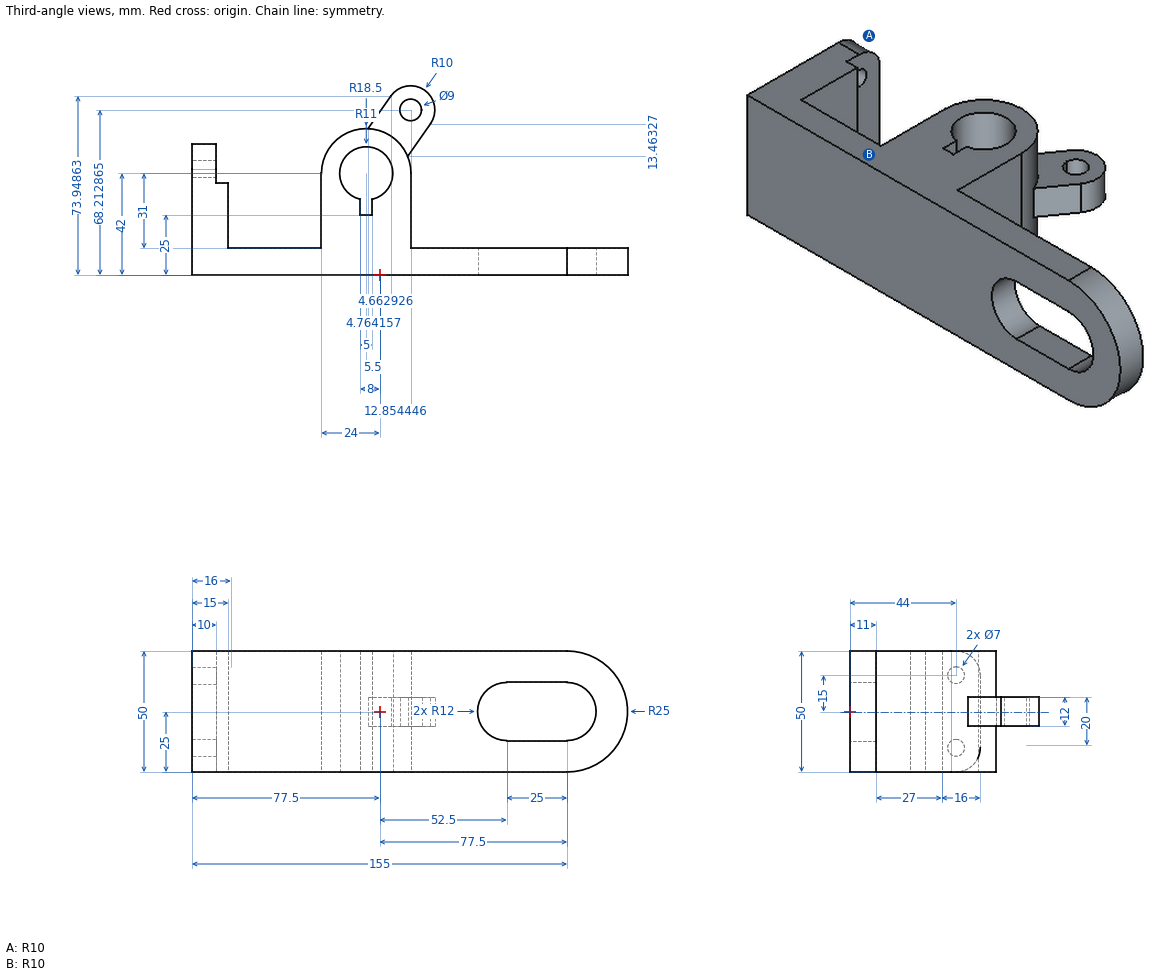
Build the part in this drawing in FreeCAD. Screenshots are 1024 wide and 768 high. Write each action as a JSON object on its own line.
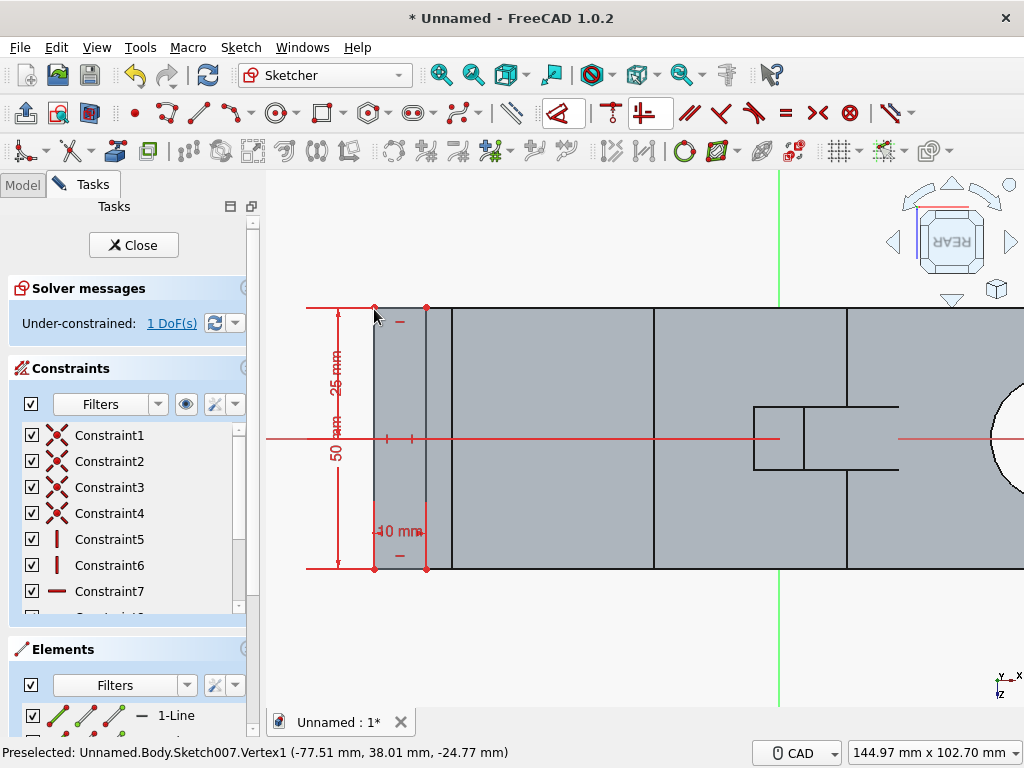
{"action": "left_click", "coordinate": [374, 308]}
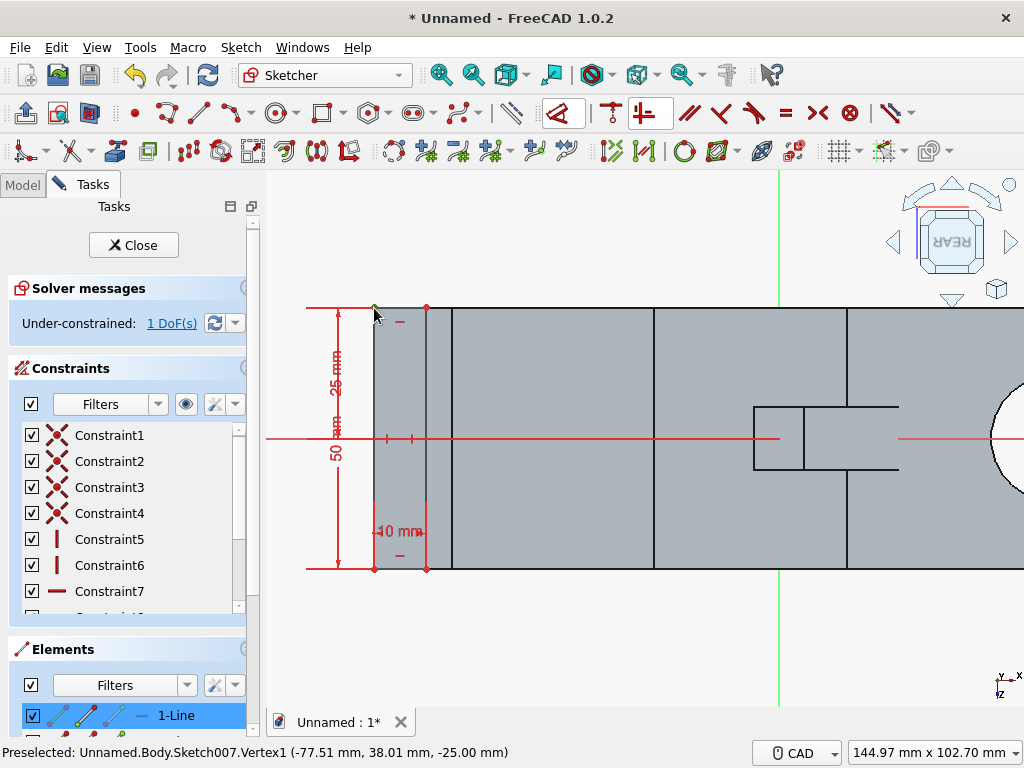
{"action": "key", "text": "l"}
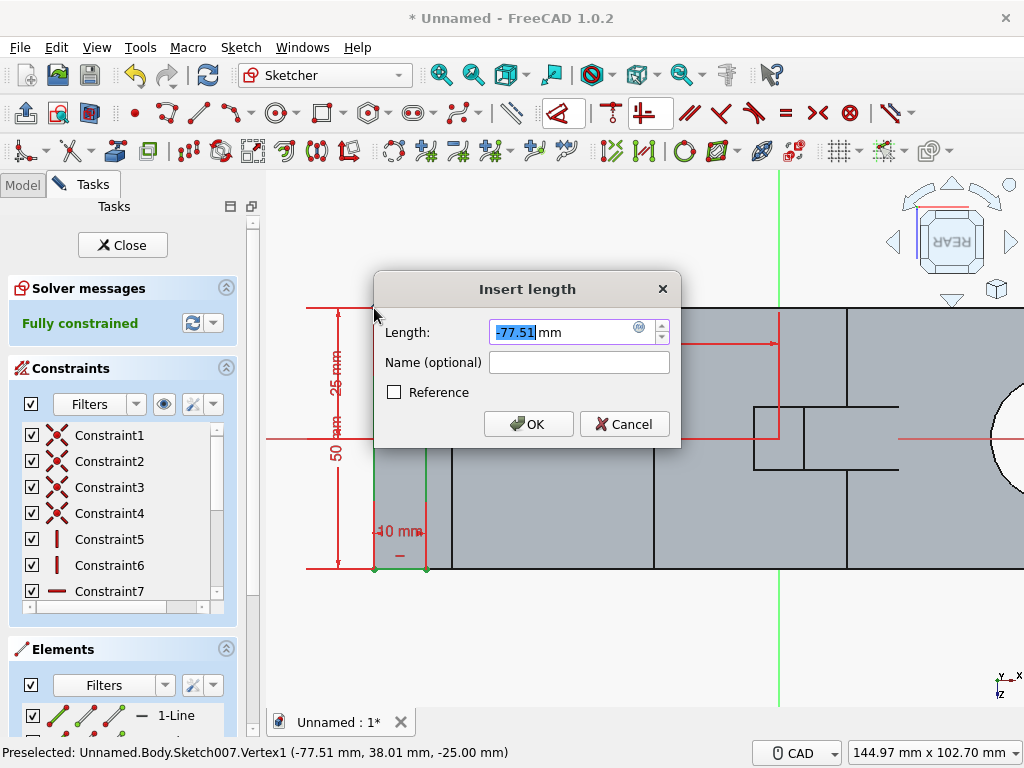
{"action": "type", "text": "-77.5"}
{"action": "key", "text": "Return"}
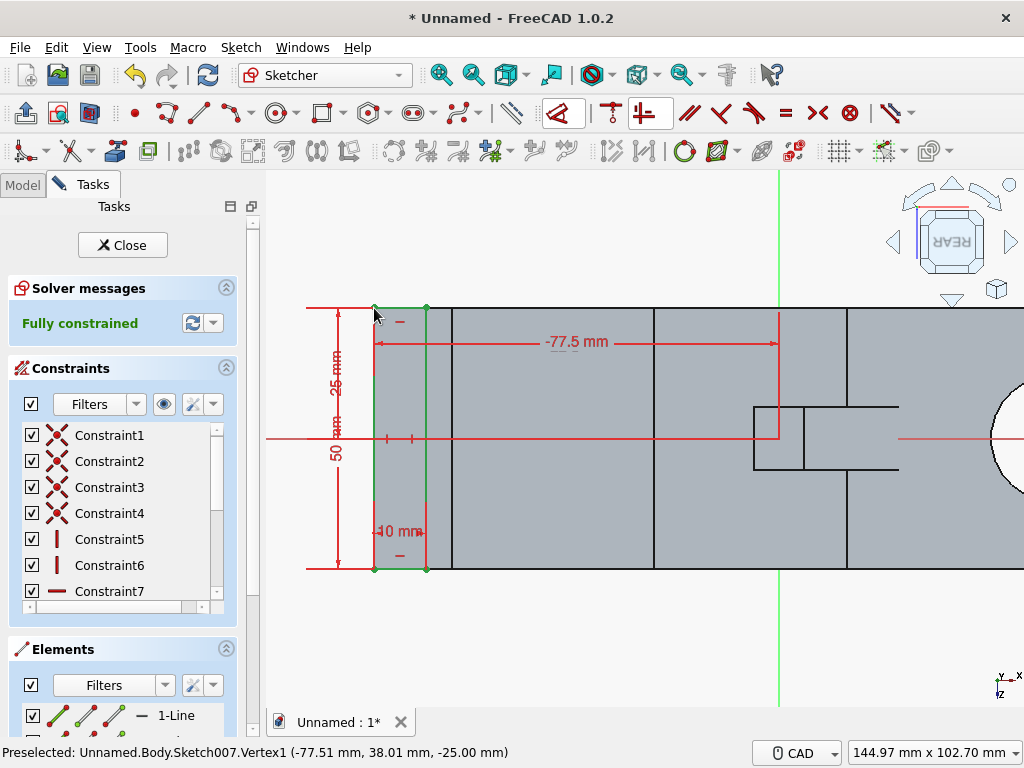
{"action": "left_click", "coordinate": [123, 245]}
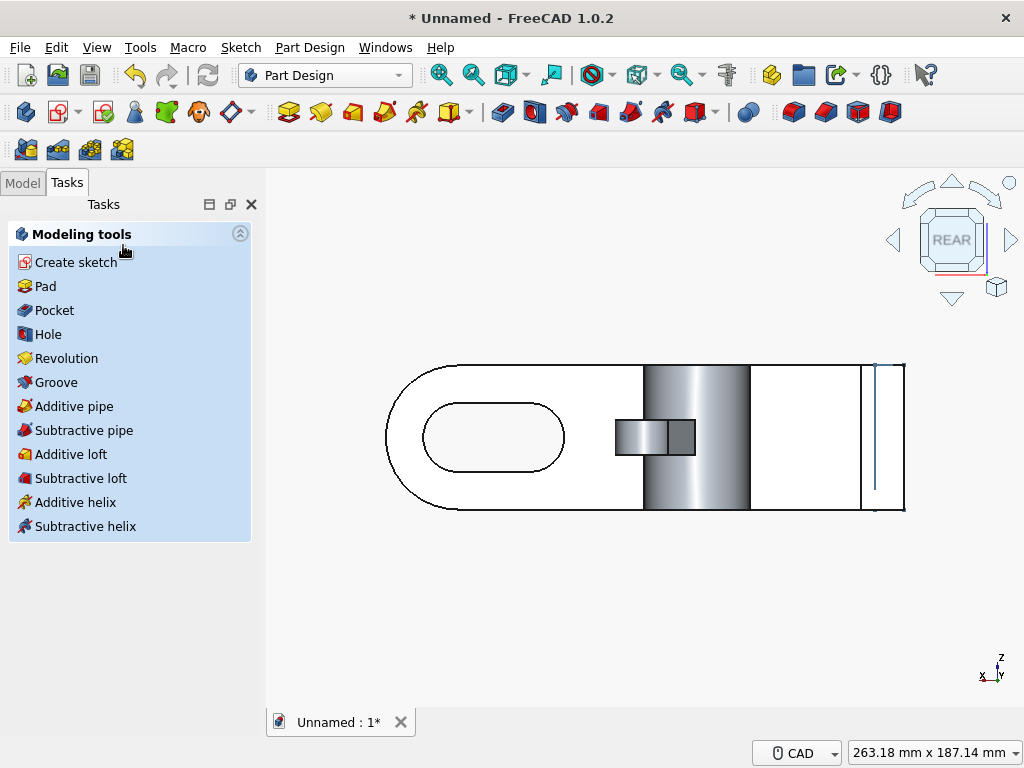
{"action": "left_click", "coordinate": [290, 112]}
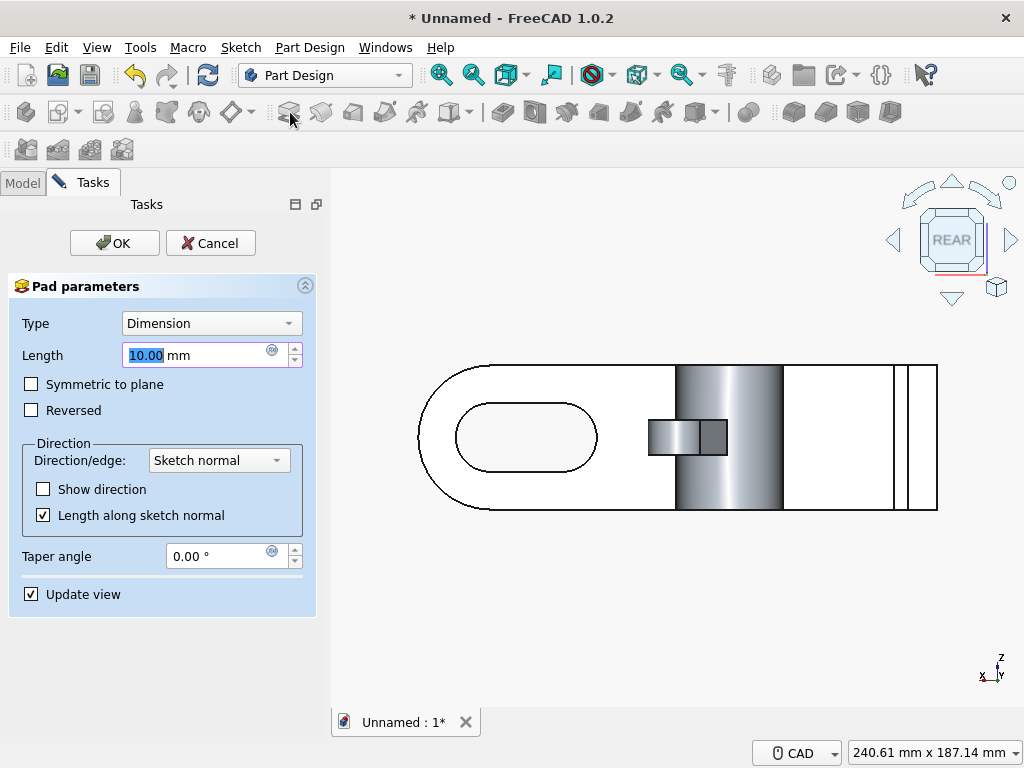
{"action": "type", "text": "16"}
{"action": "key", "text": "Tab"}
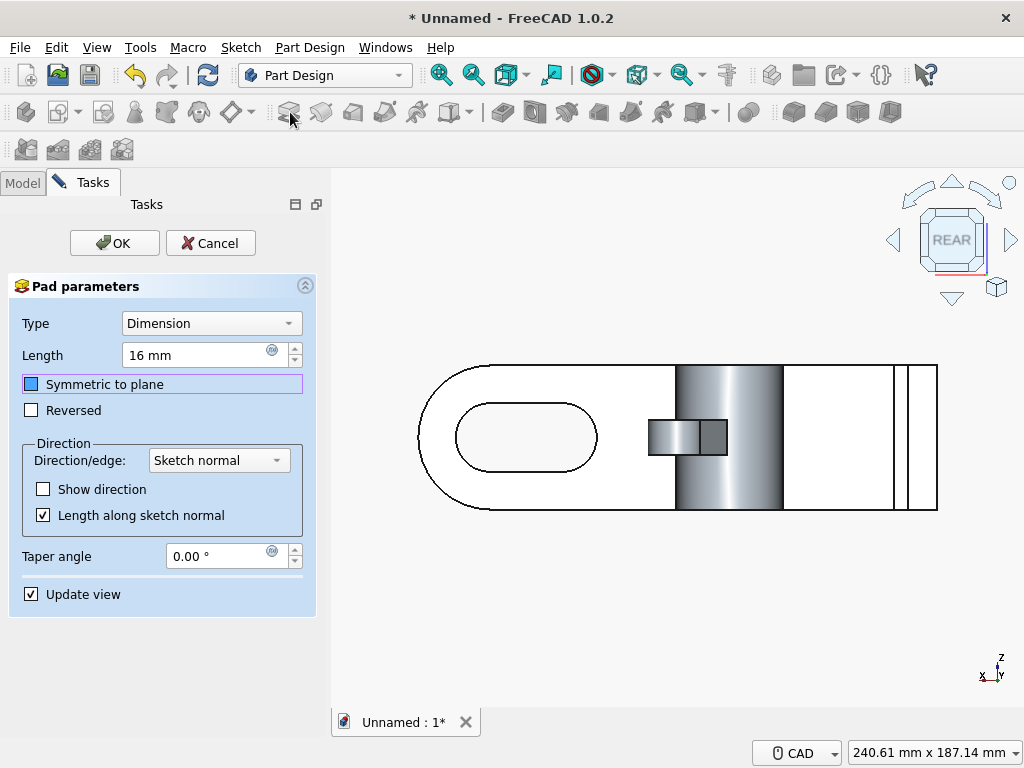
{"action": "left_click", "coordinate": [115, 243]}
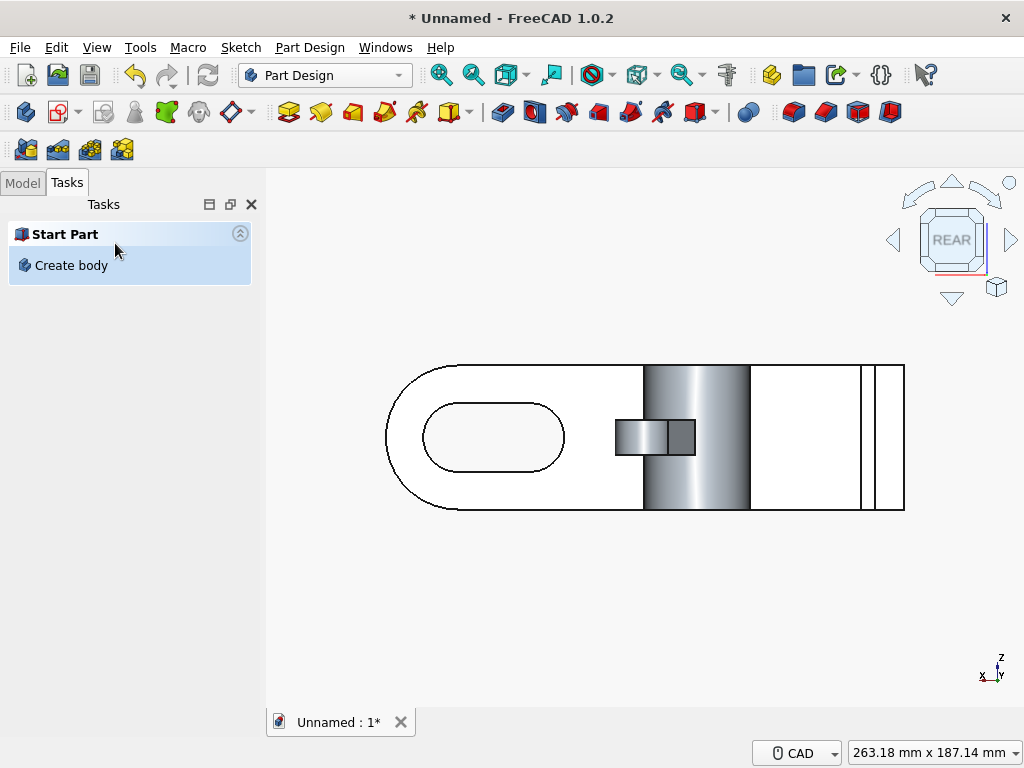
{"action": "key", "text": "0"}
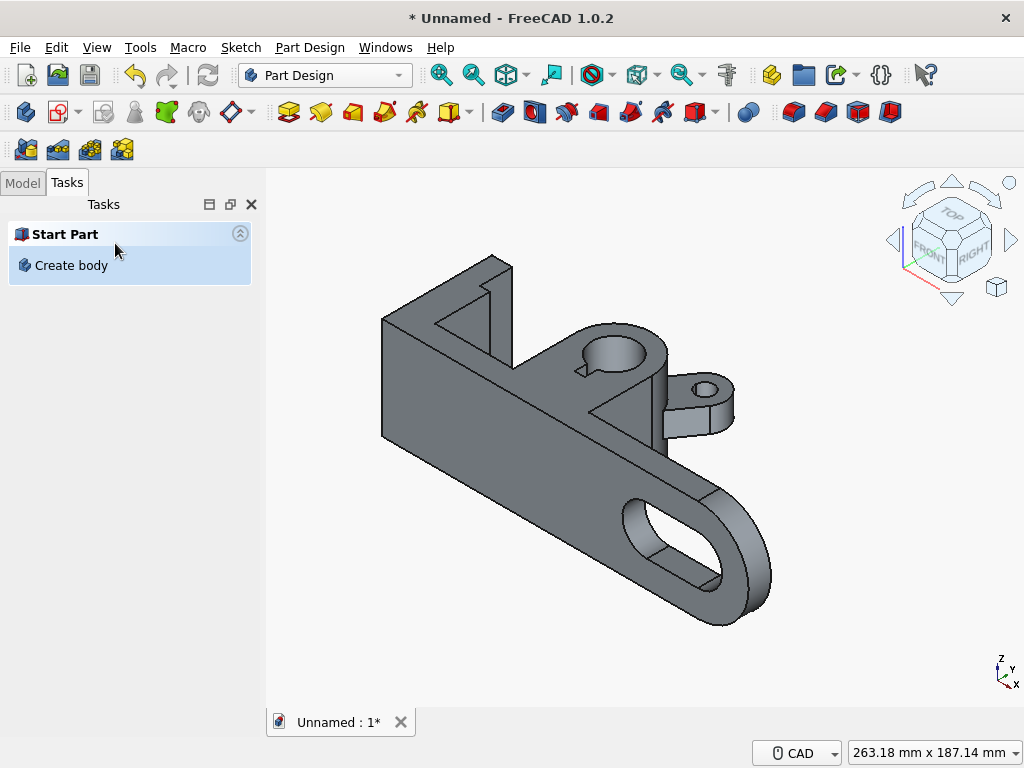
{"action": "key", "text": "2"}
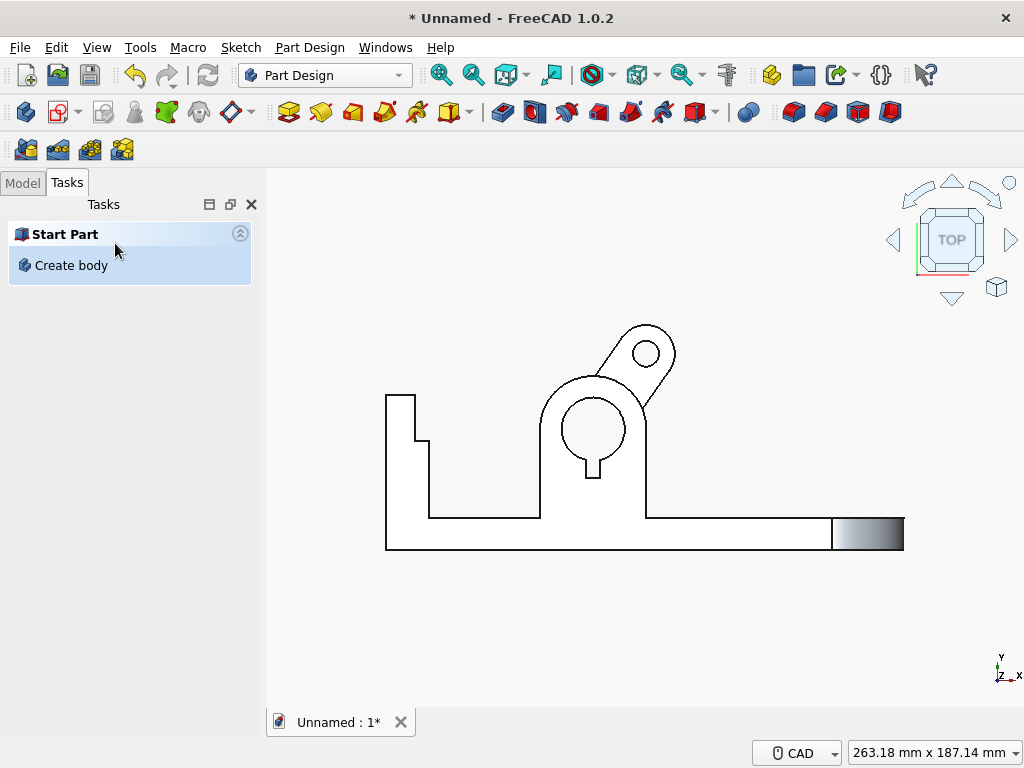
{"action": "left_click", "coordinate": [400, 394]}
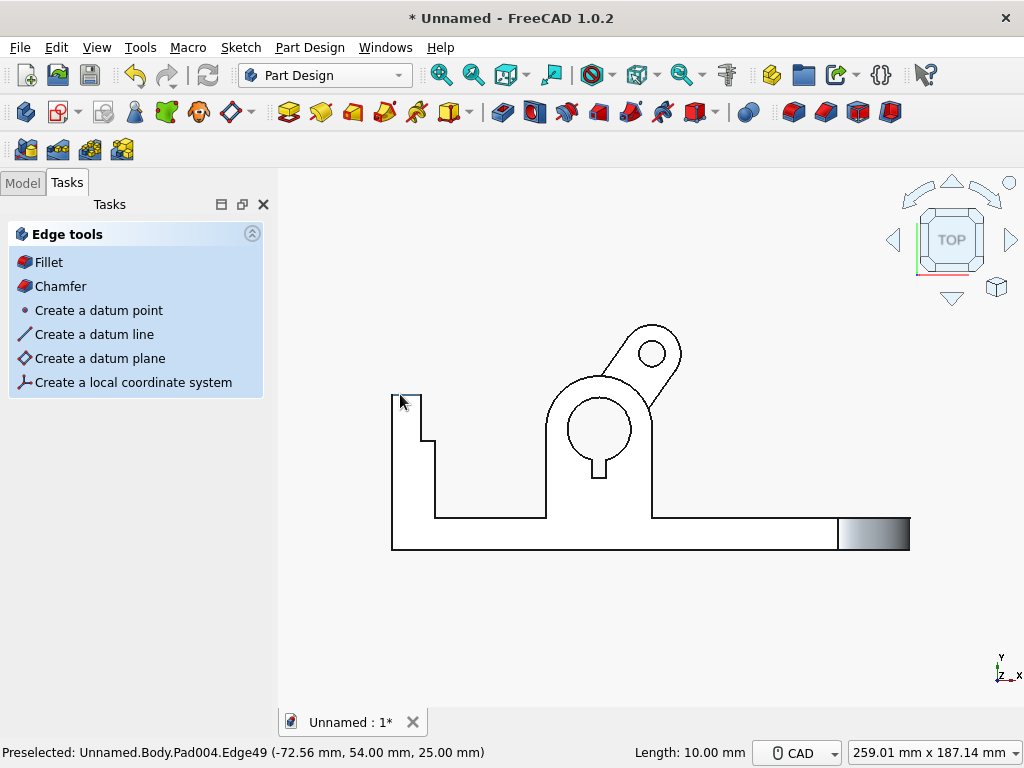
{"action": "left_click", "coordinate": [794, 112]}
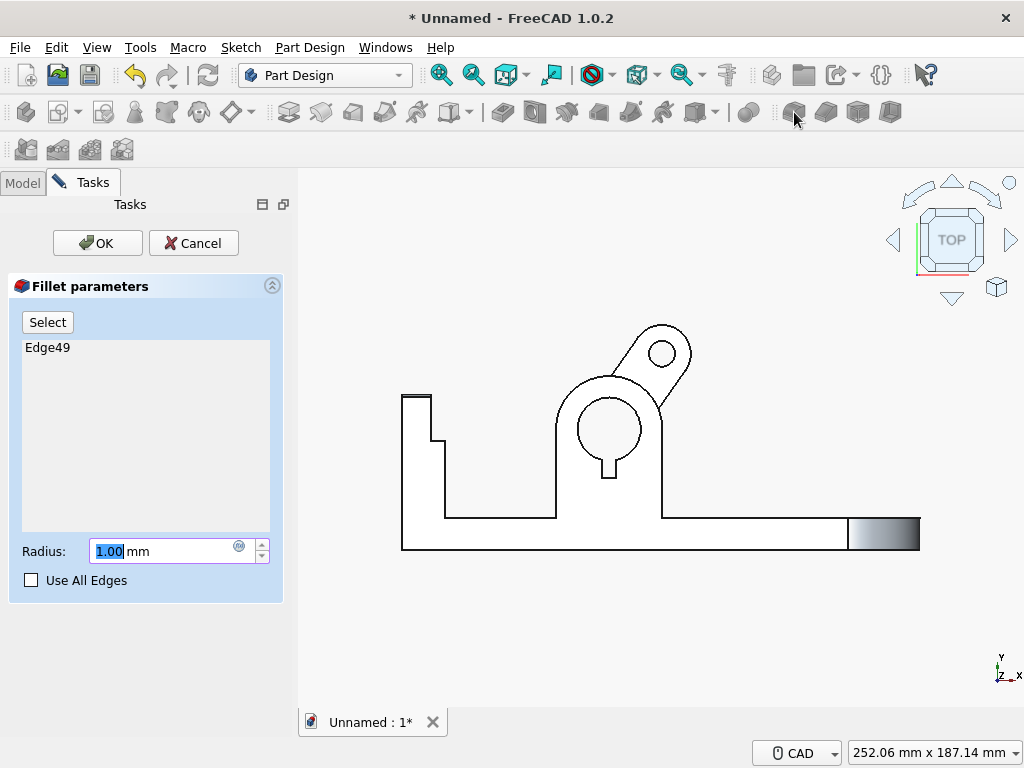
{"action": "type", "text": "10"}
{"action": "key", "text": "Tab"}